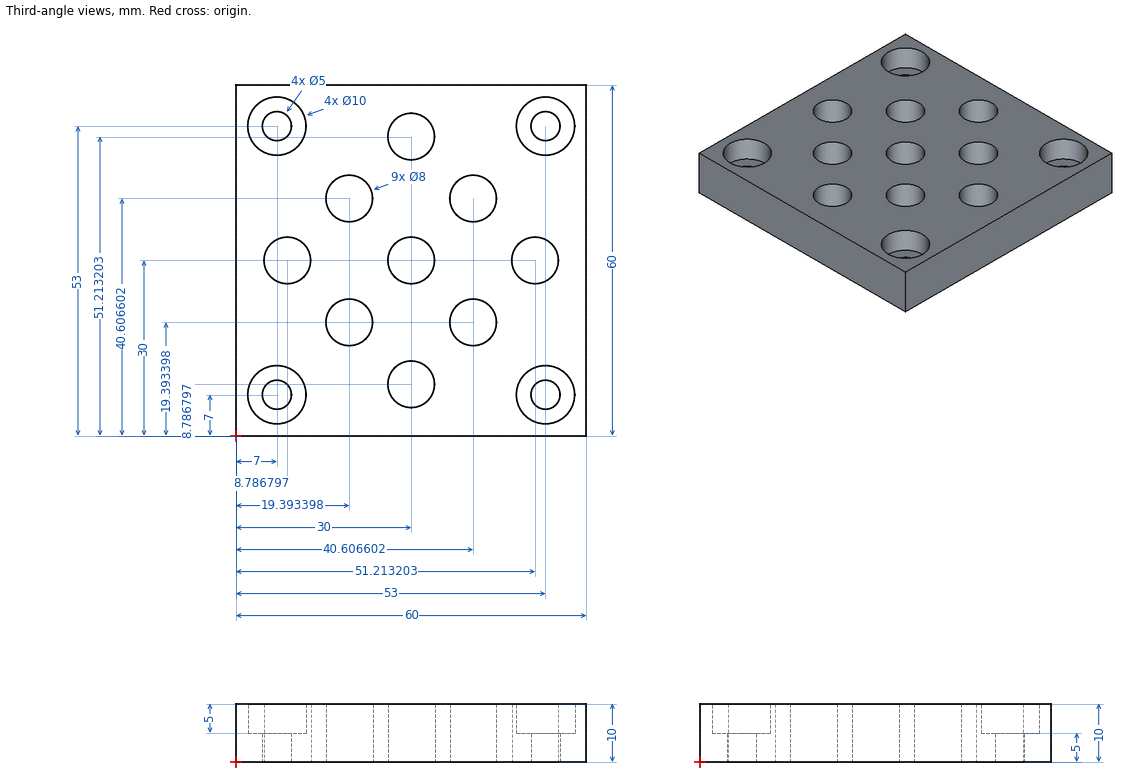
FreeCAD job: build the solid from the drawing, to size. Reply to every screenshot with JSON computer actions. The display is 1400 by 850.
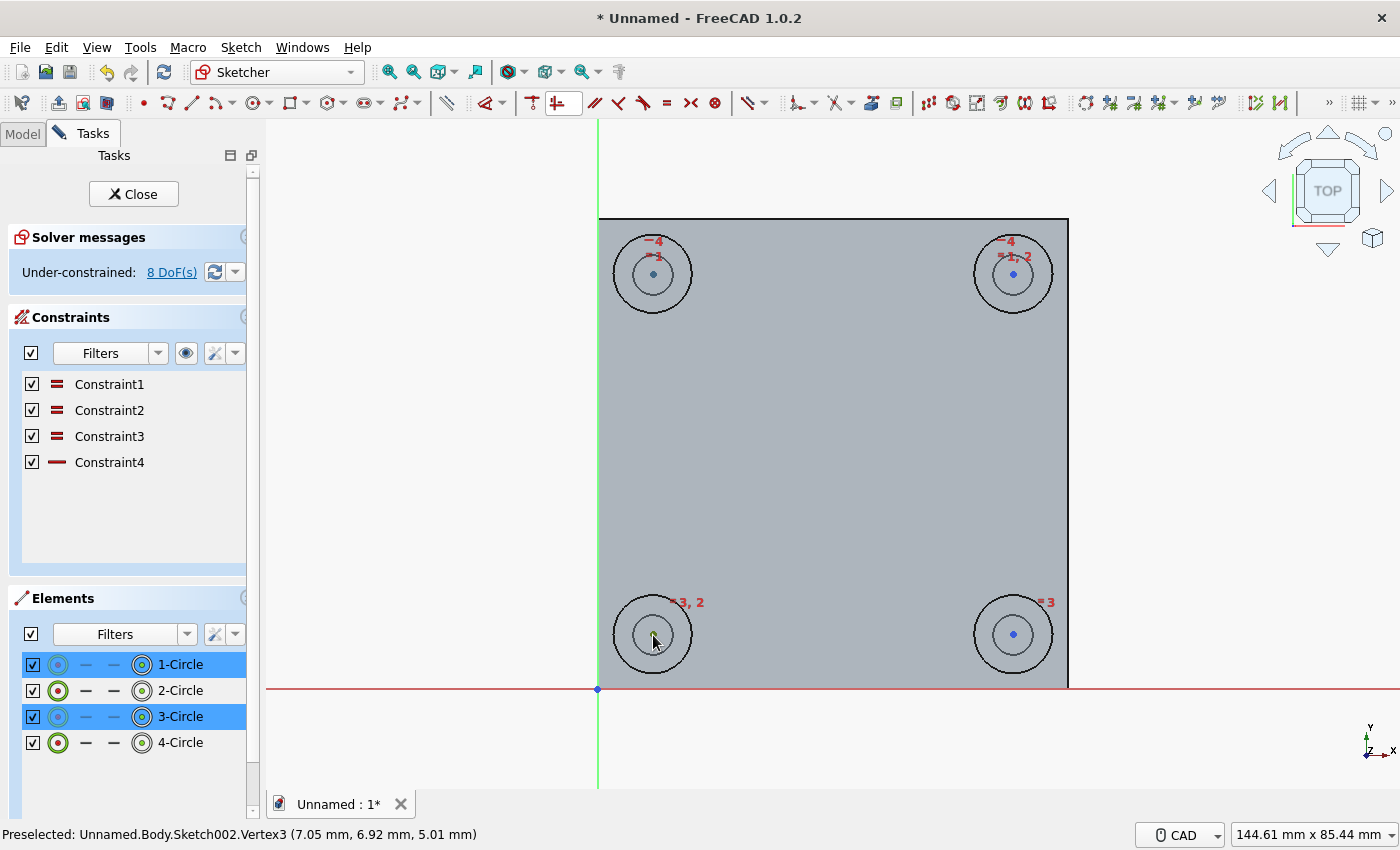
{"action": "key", "text": "v"}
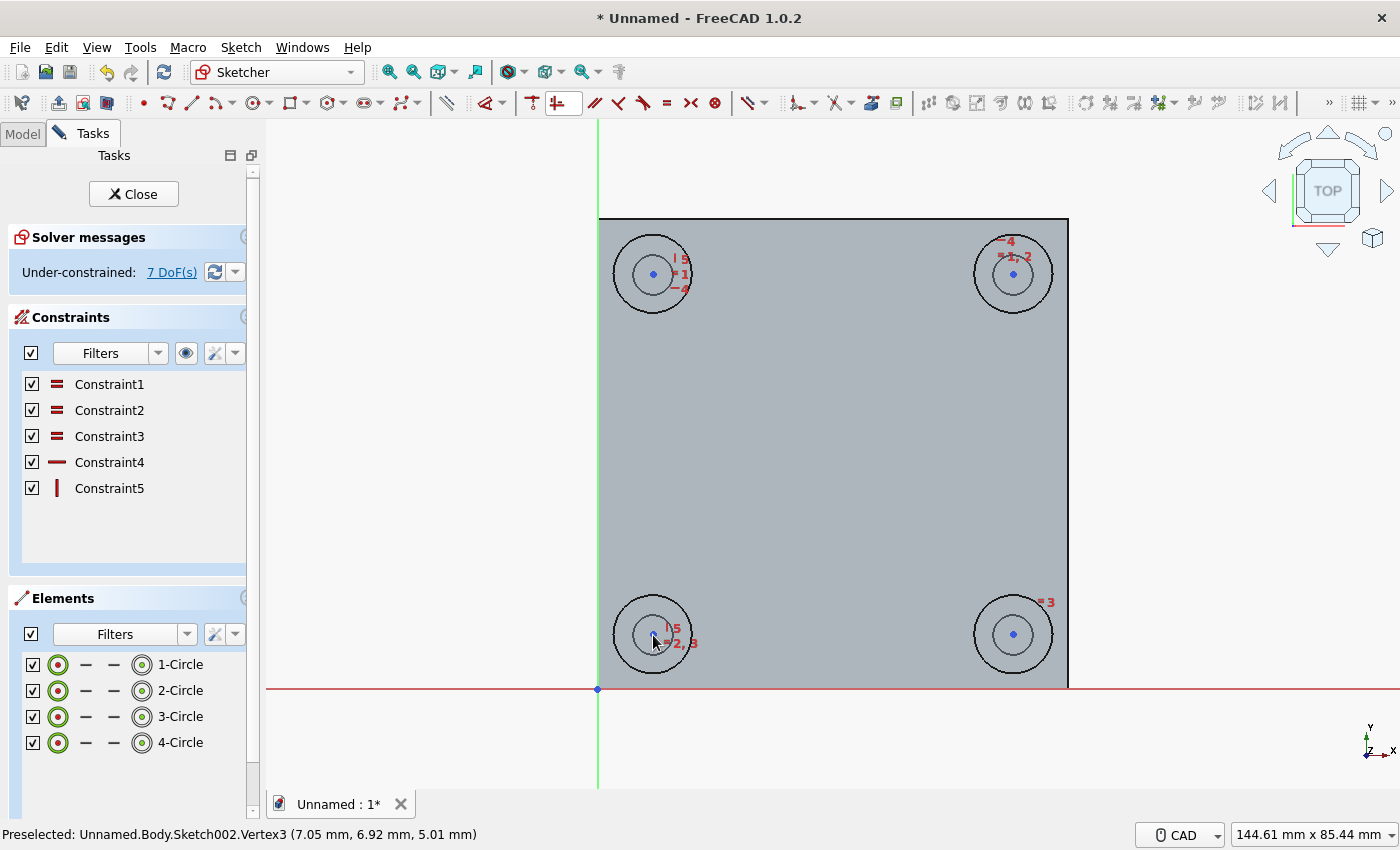
{"action": "left_click", "coordinate": [1013, 275]}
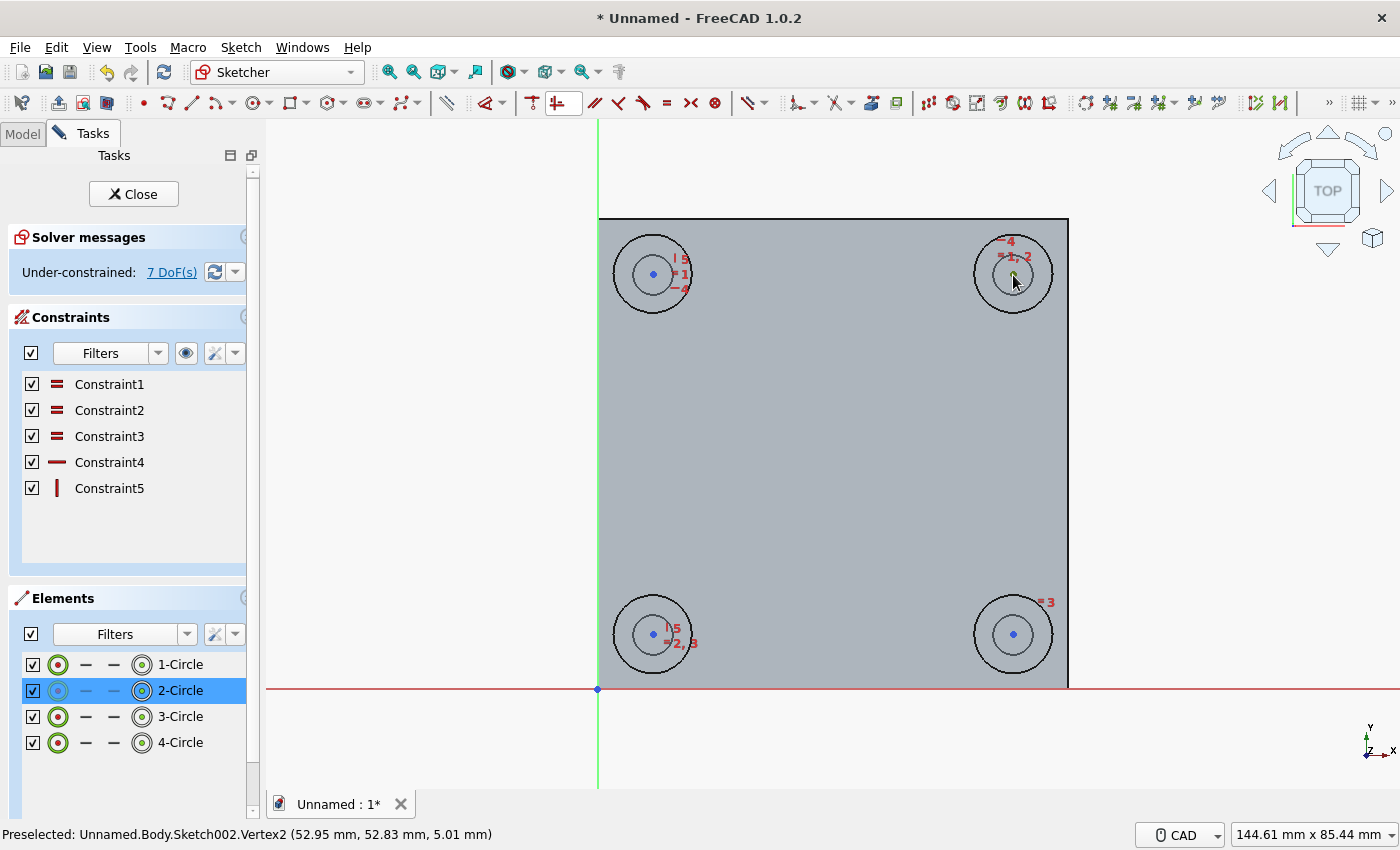
{"action": "left_click", "coordinate": [1013, 635]}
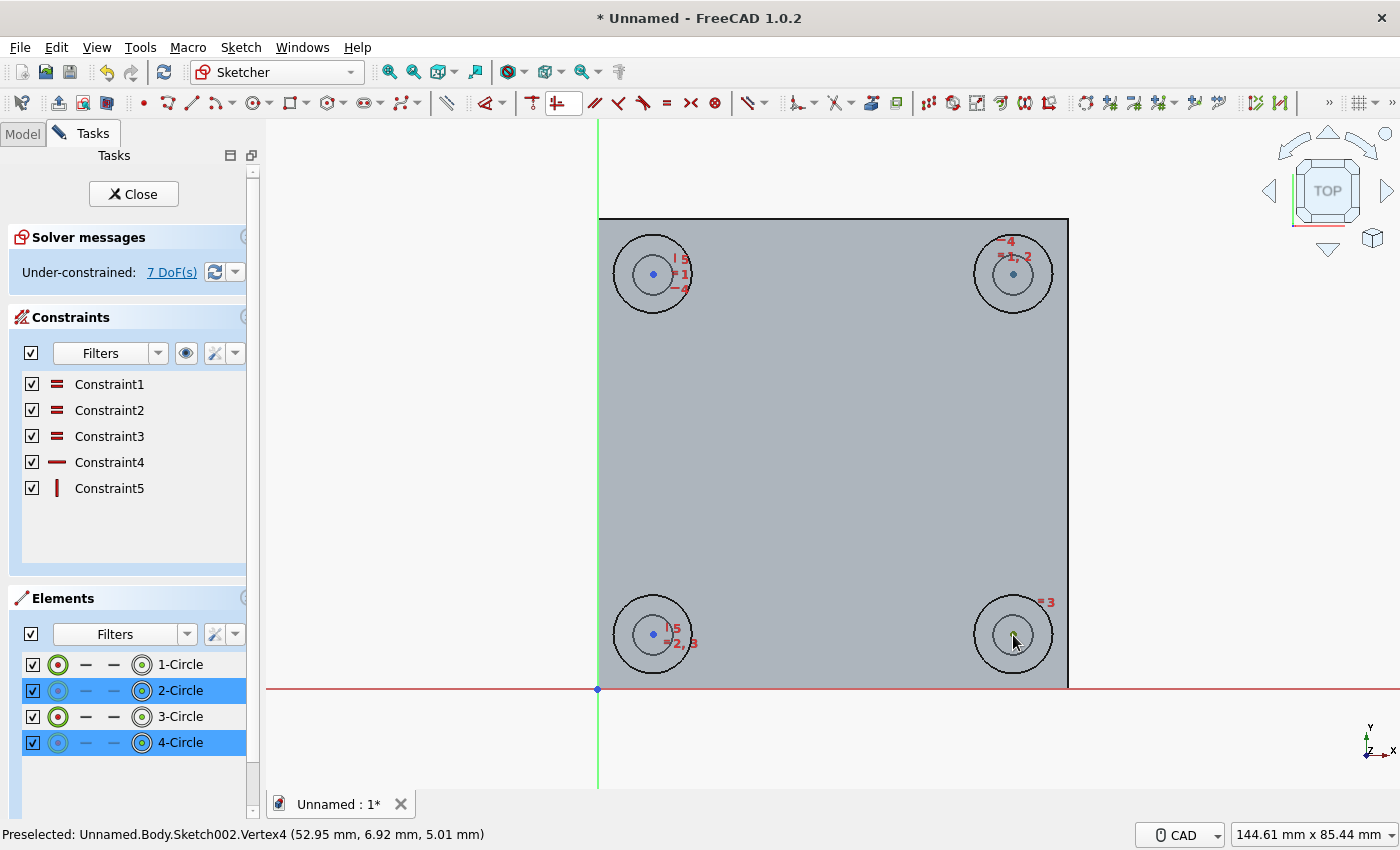
{"action": "left_click", "coordinate": [576, 104]}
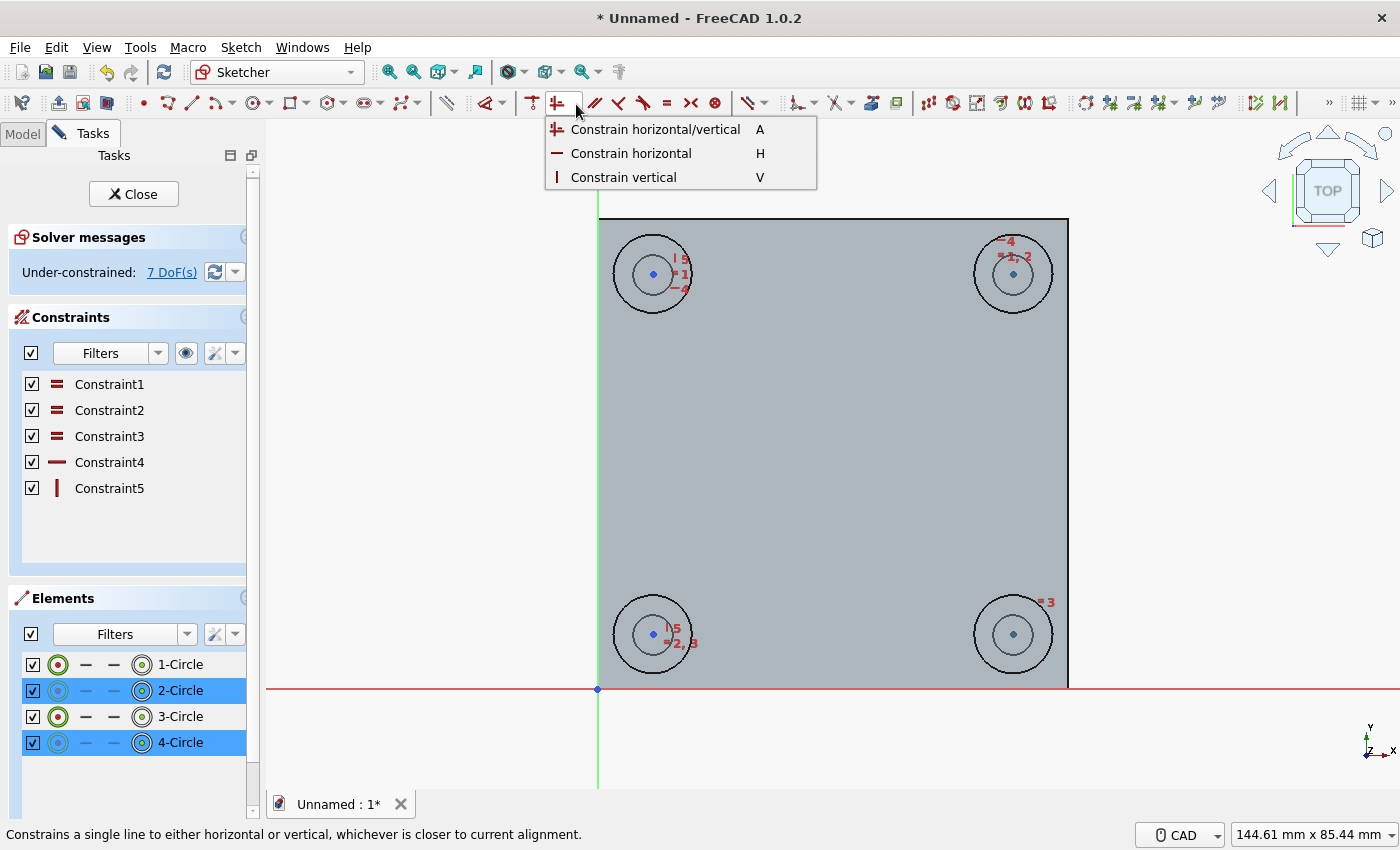
{"action": "left_click", "coordinate": [681, 177]}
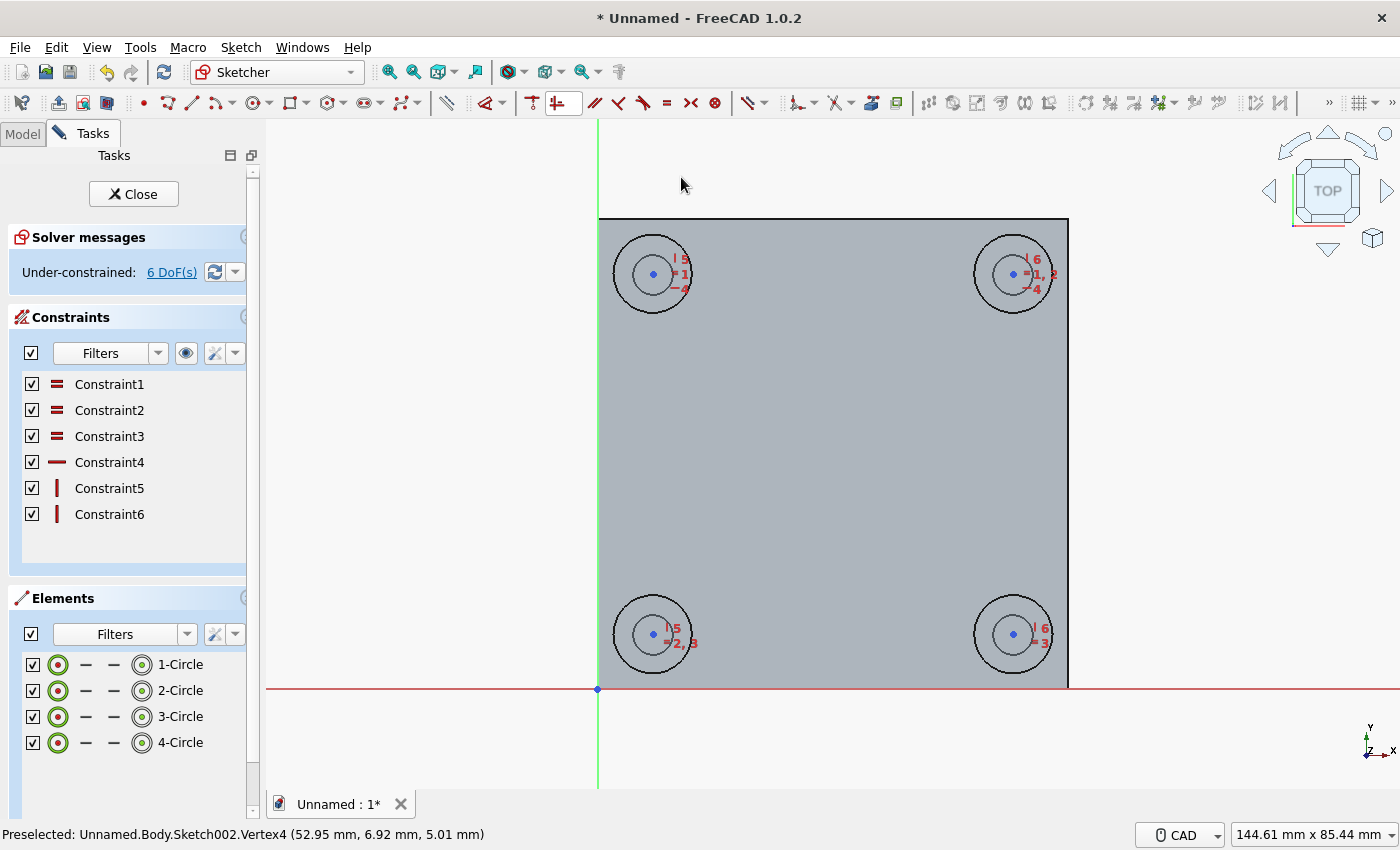
{"action": "left_click", "coordinate": [653, 635]}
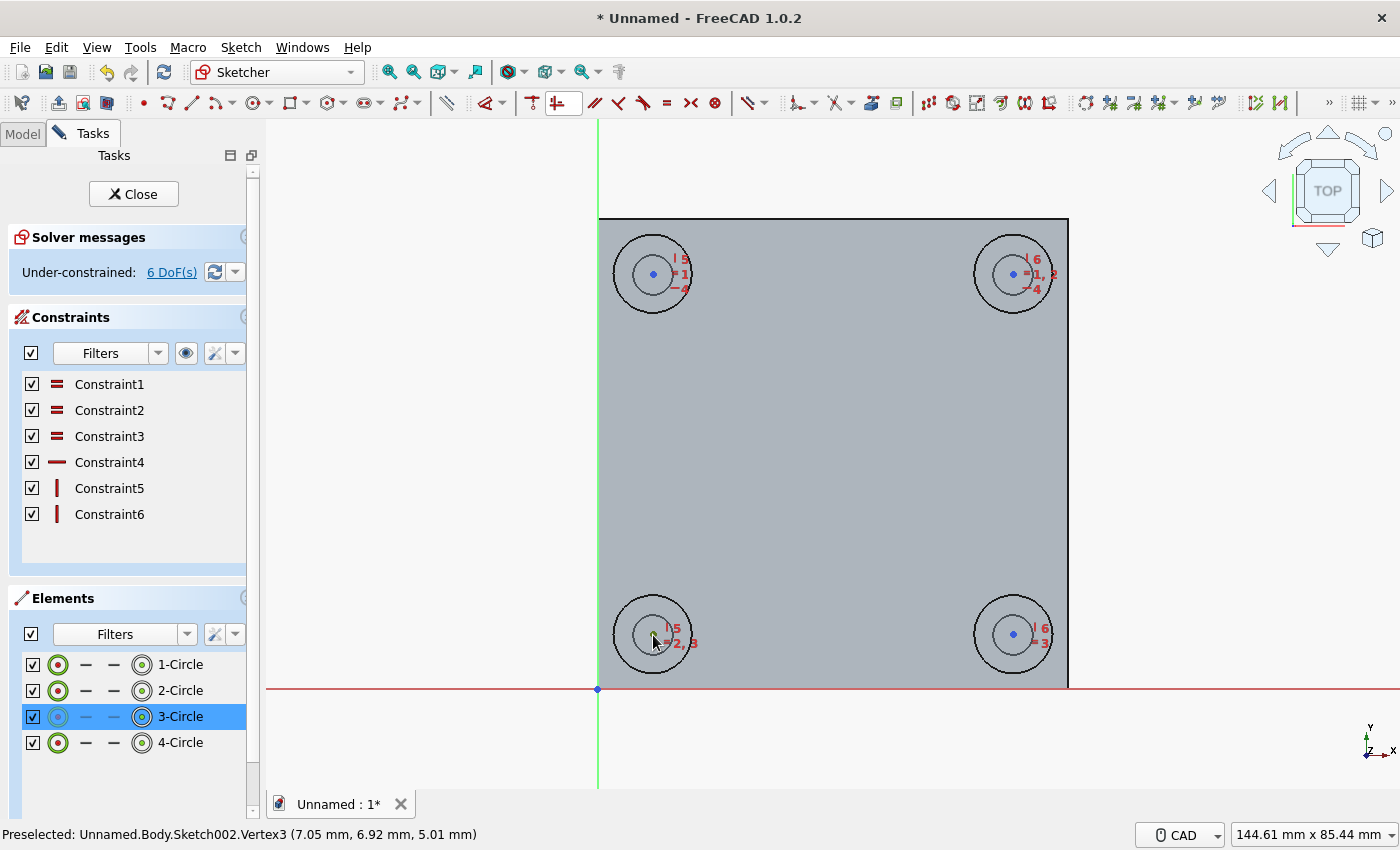
{"action": "left_click", "coordinate": [1013, 635]}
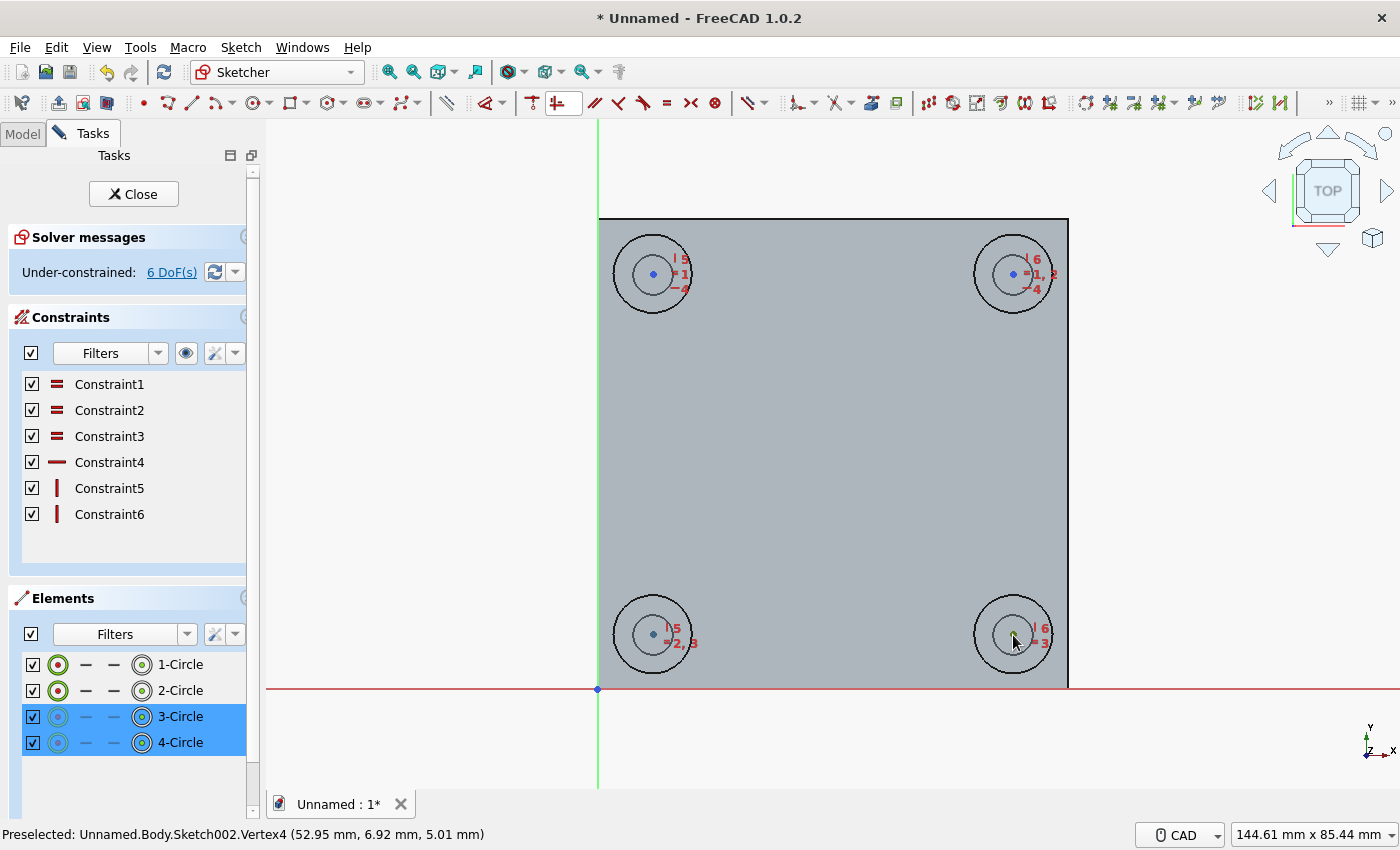
{"action": "key", "text": "h"}